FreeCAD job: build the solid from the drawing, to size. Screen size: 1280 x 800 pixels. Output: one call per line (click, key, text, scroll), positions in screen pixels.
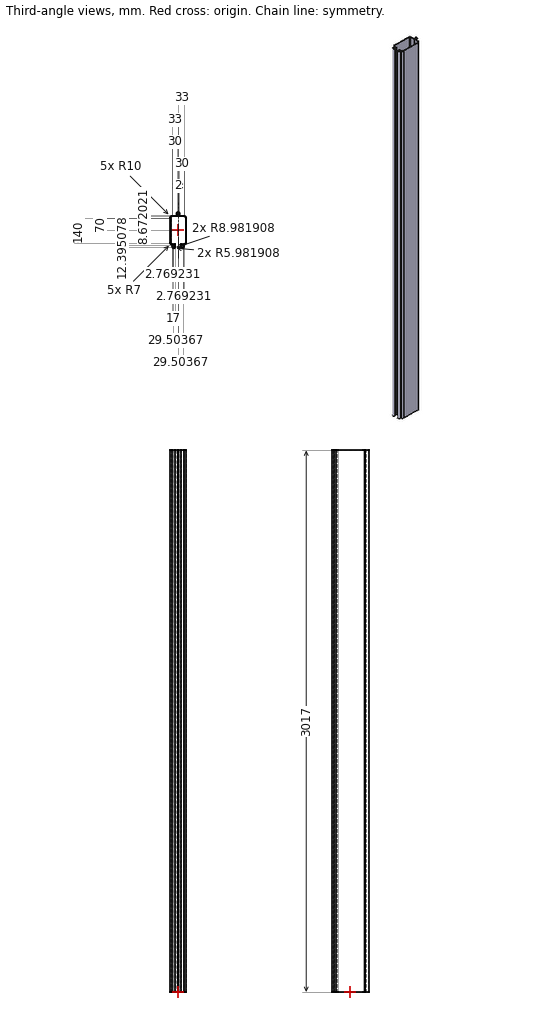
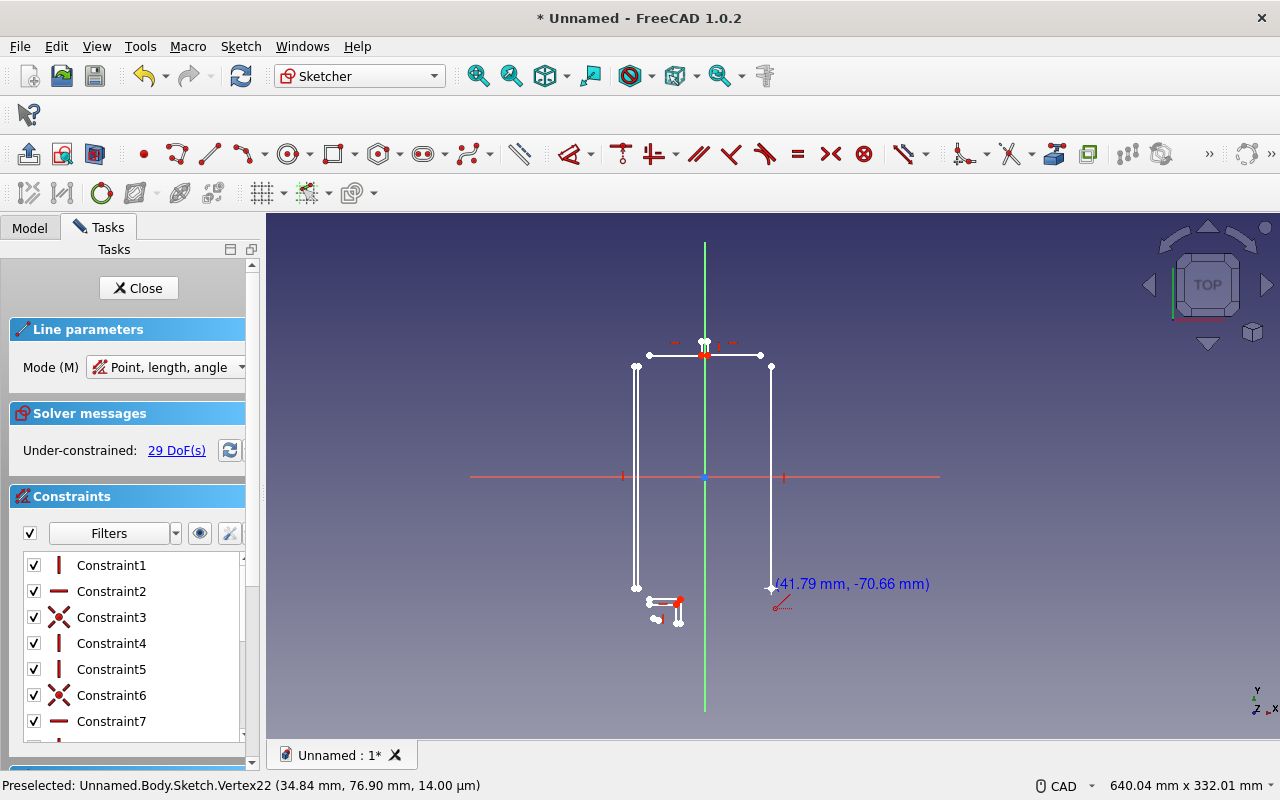
click(177, 154)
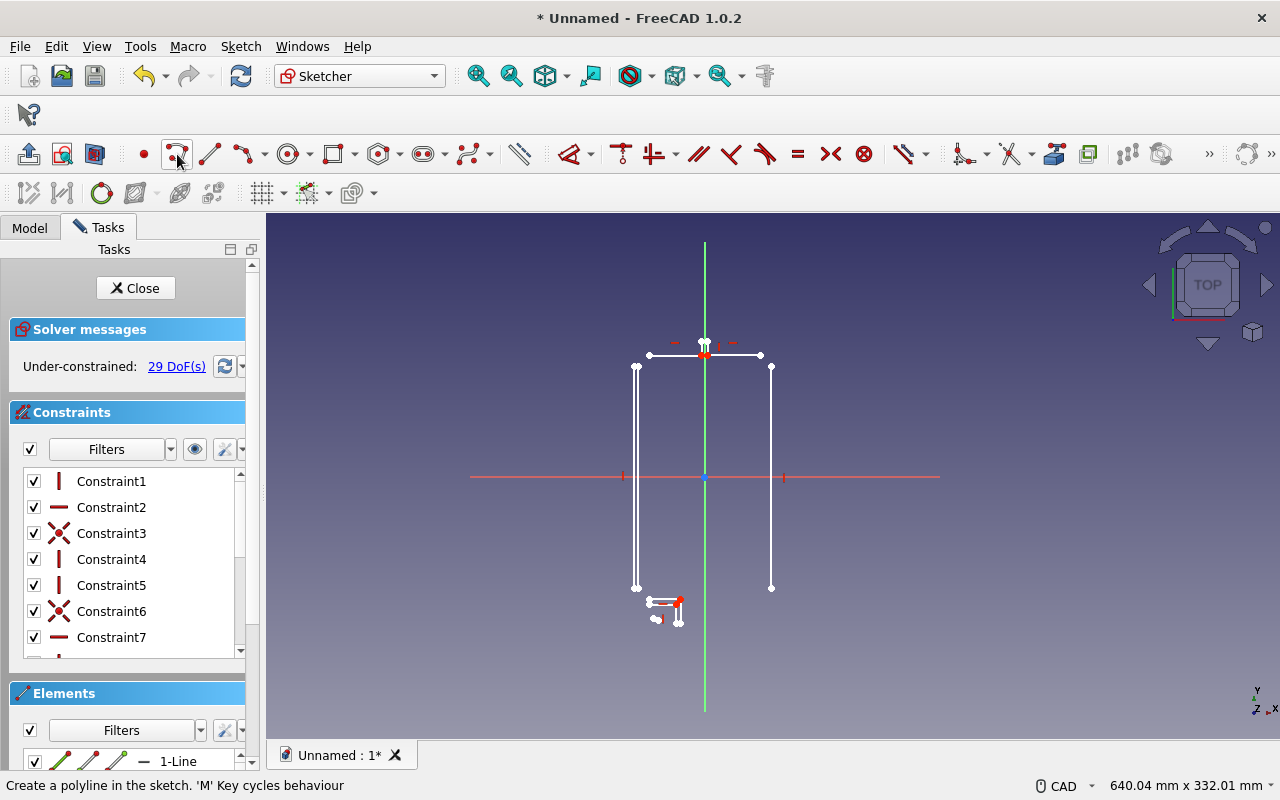
click(760, 599)
click(729, 599)
click(729, 623)
right_click(729, 623)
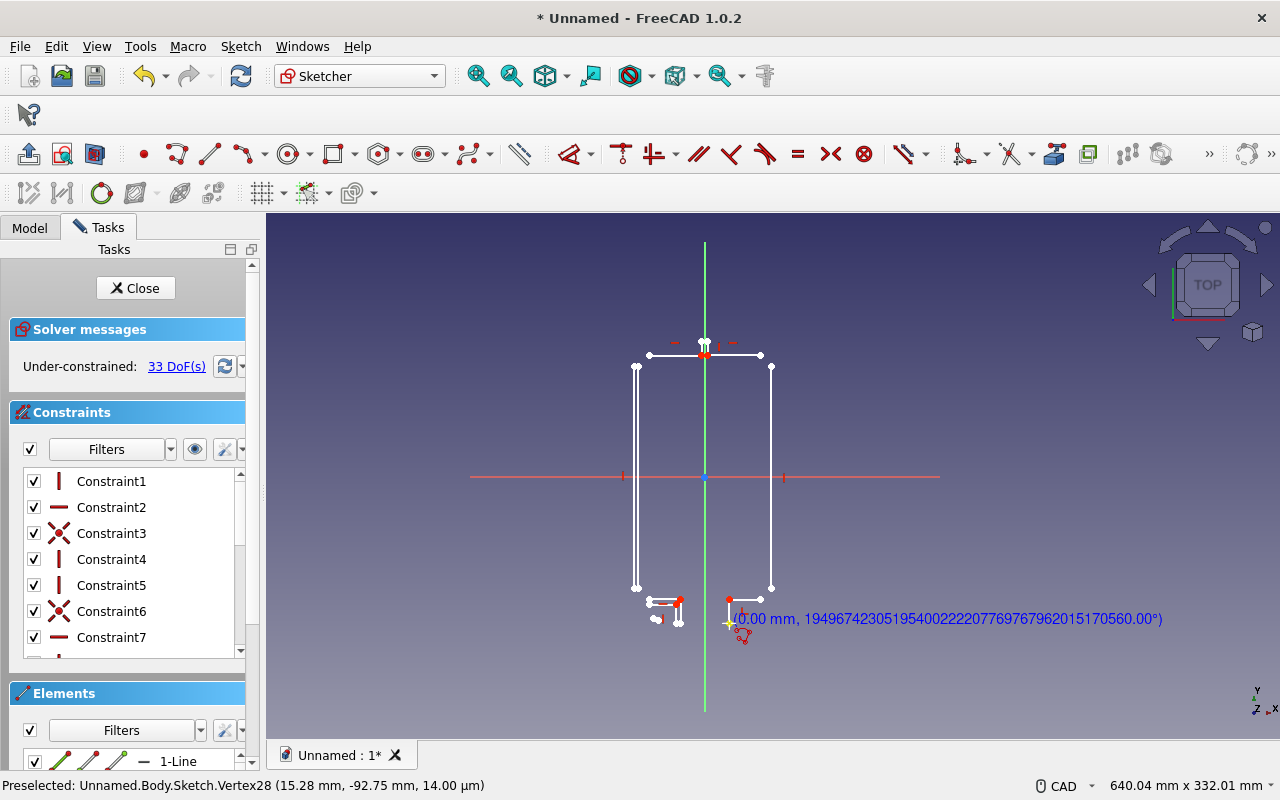
click(210, 154)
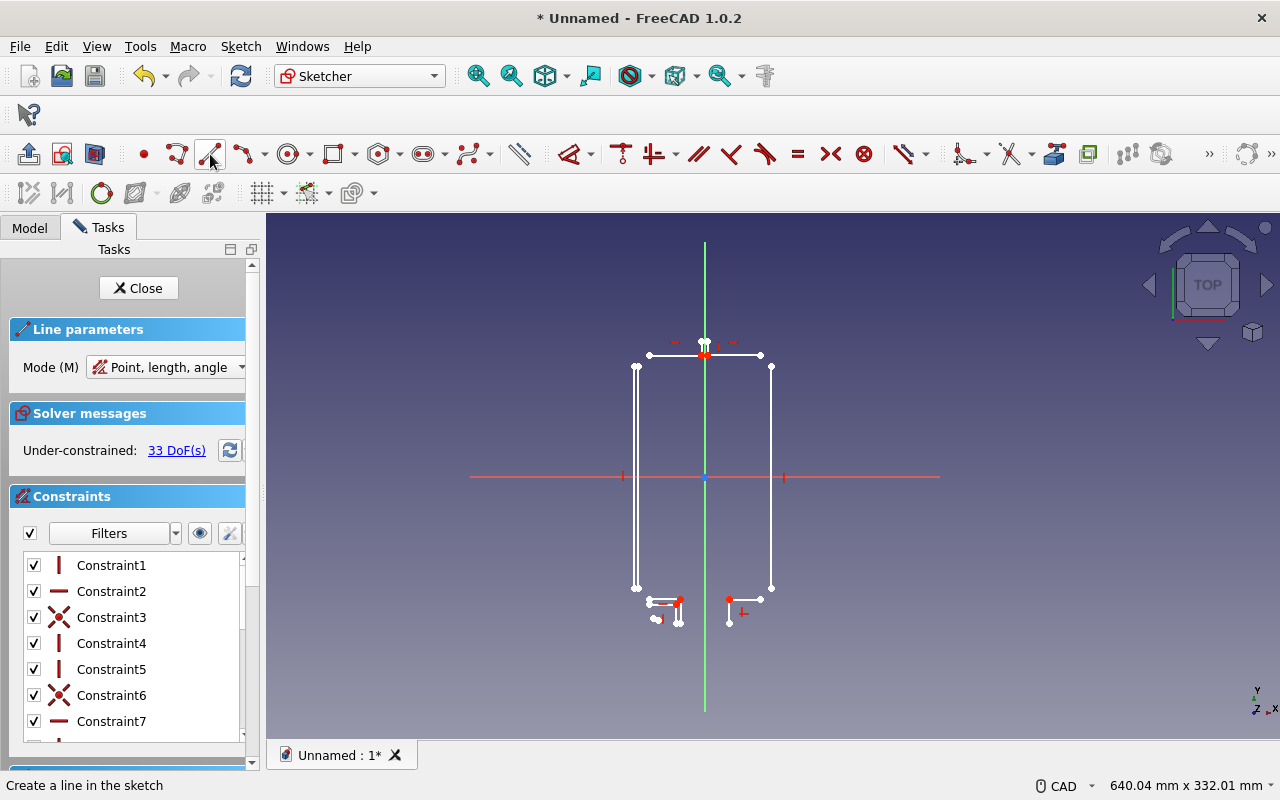
click(756, 618)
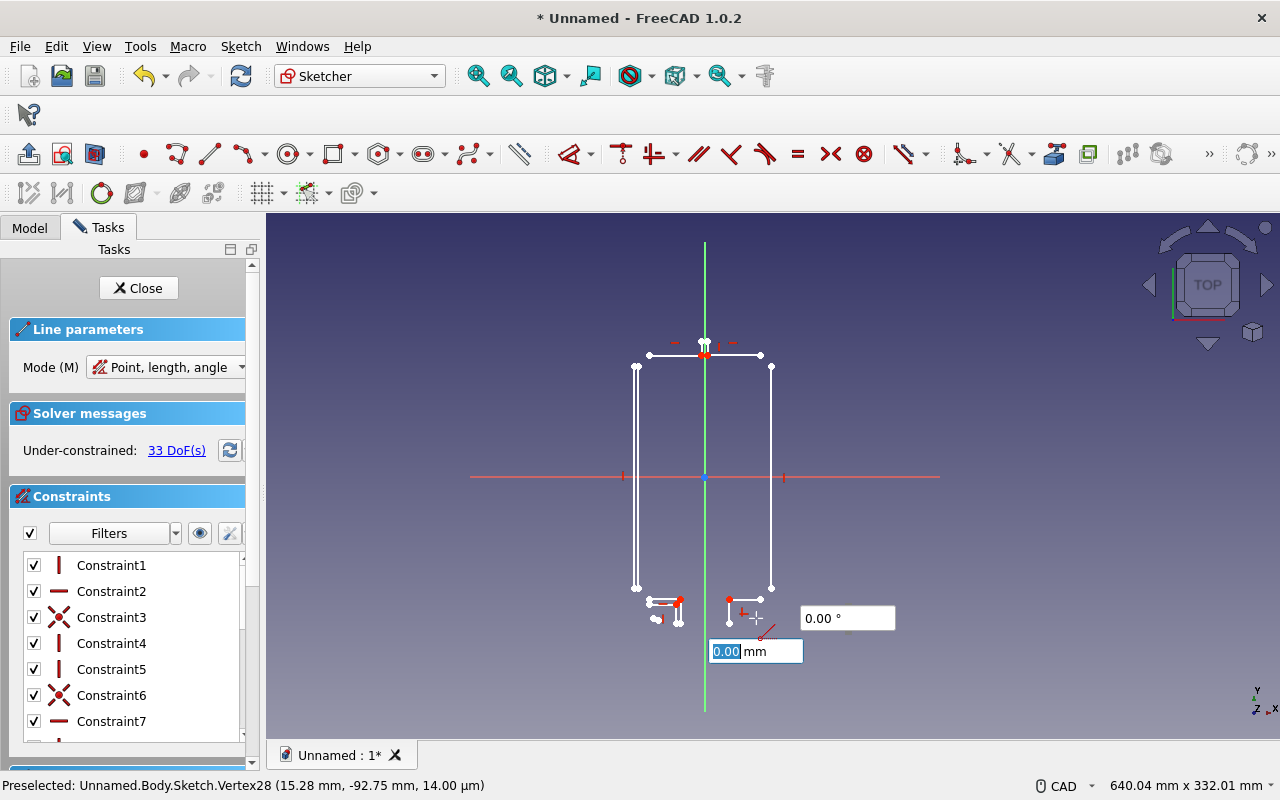
scroll(752, 620, up, 7)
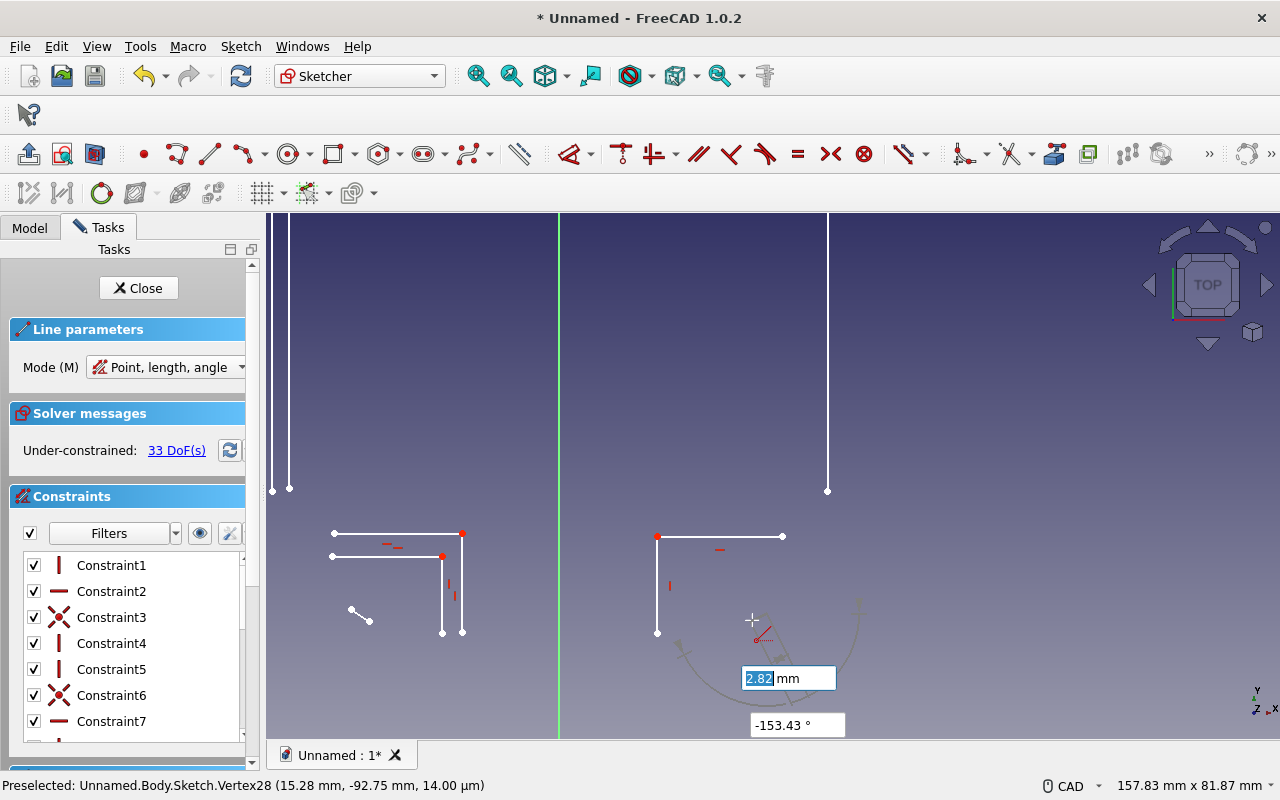
click(749, 617)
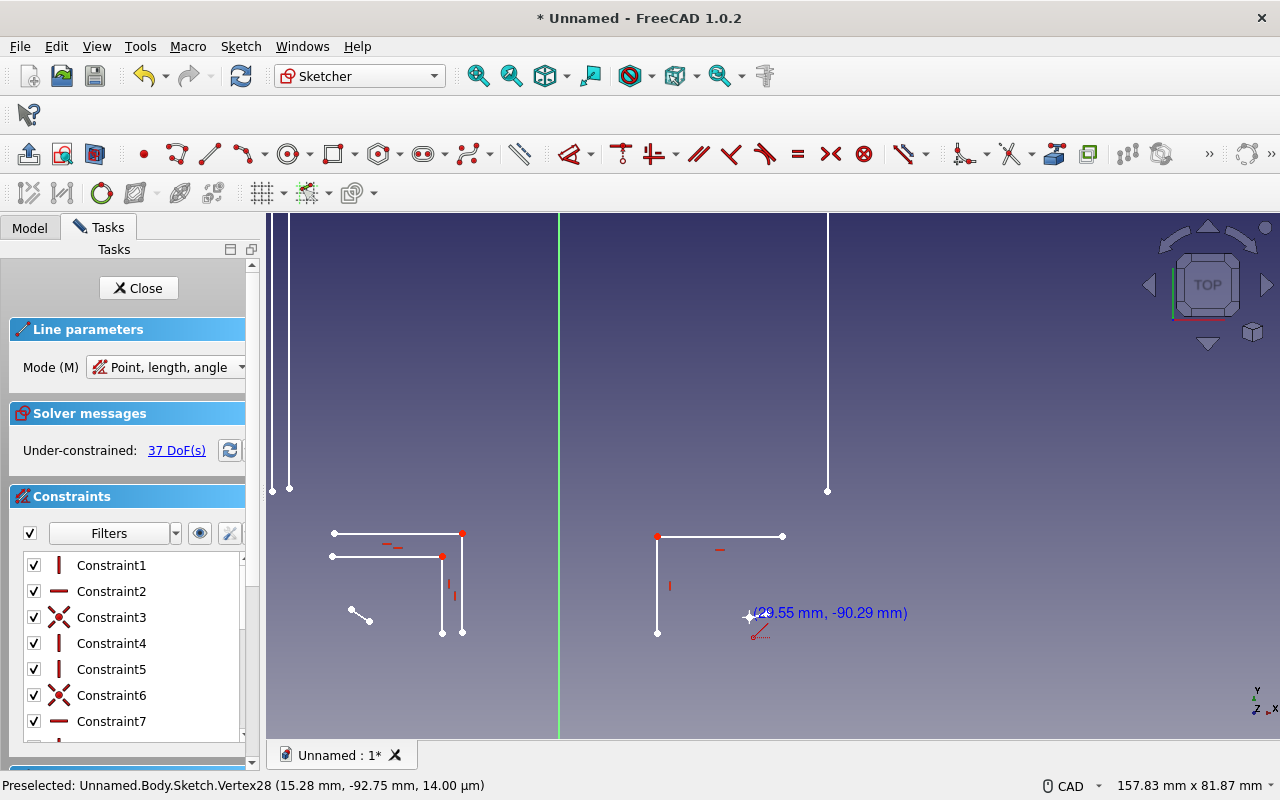
click(177, 154)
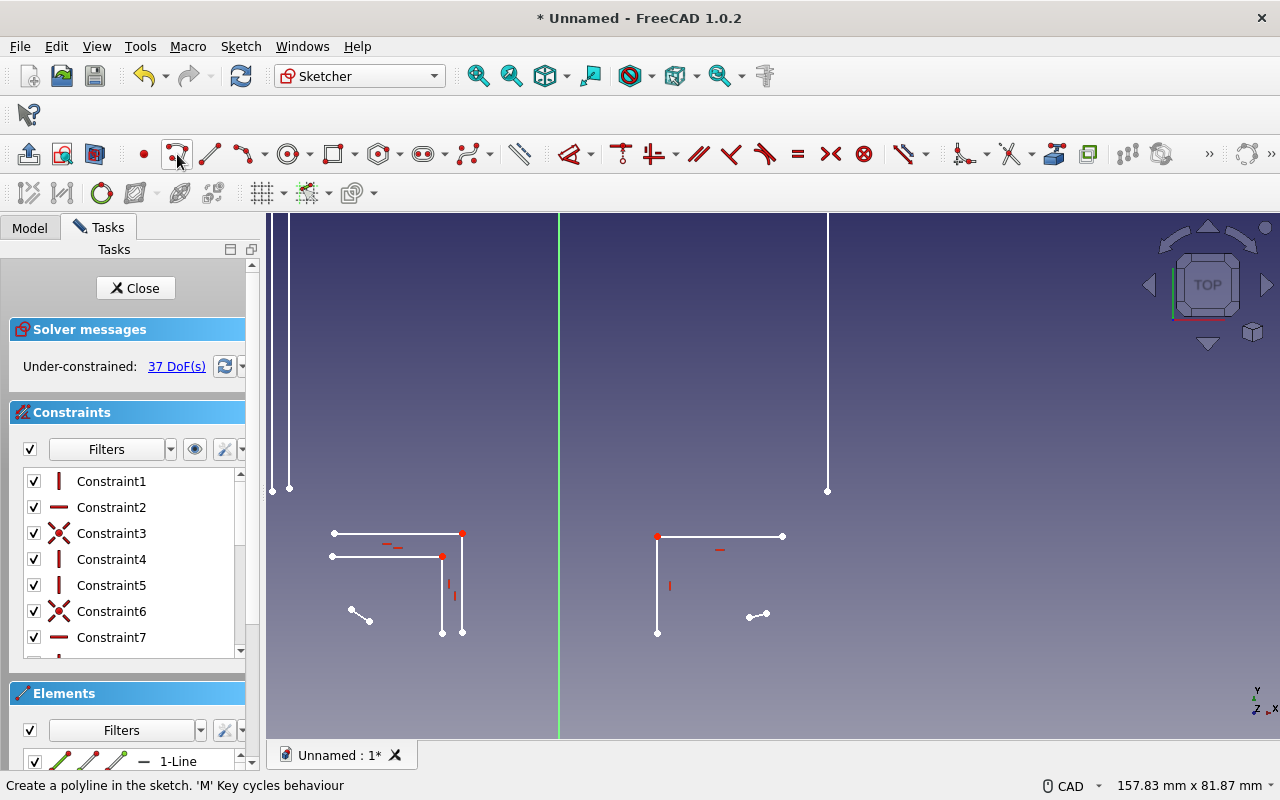
click(675, 632)
click(675, 552)
click(784, 552)
right_click(784, 552)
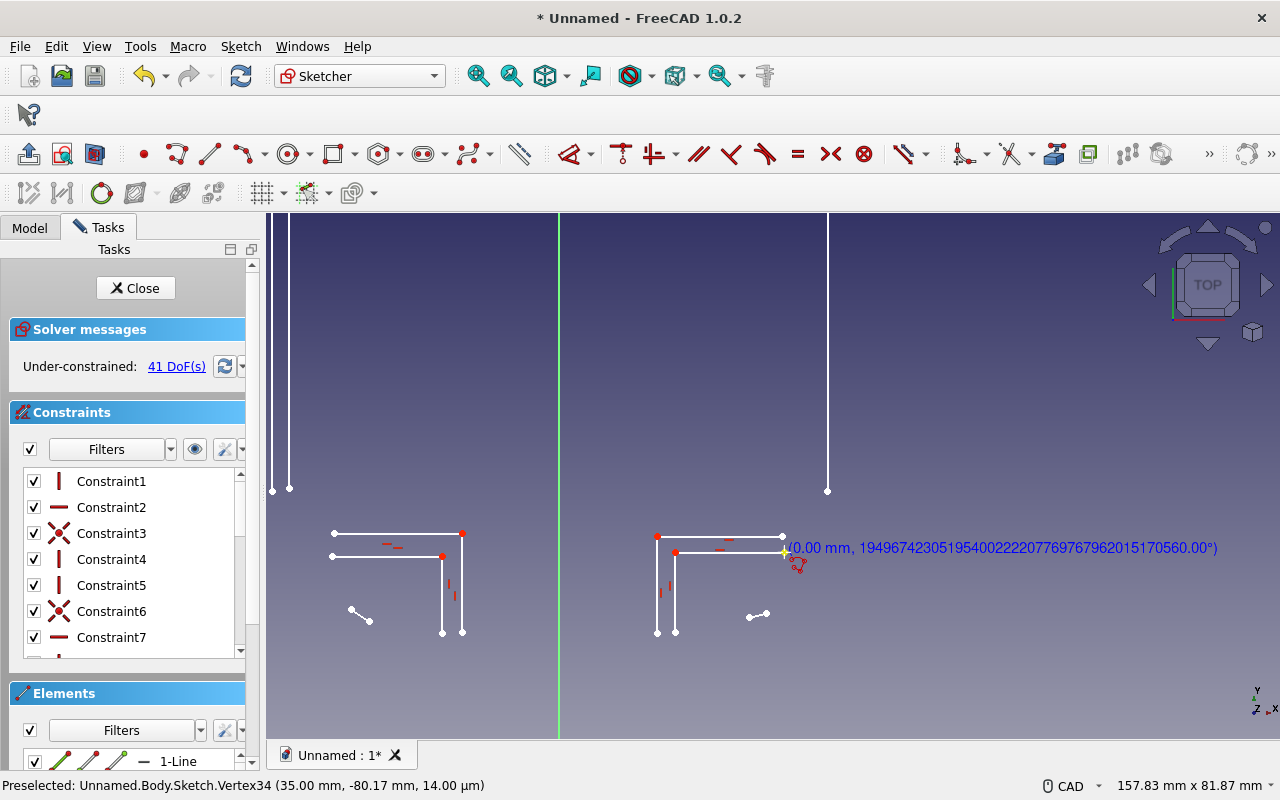
click(210, 154)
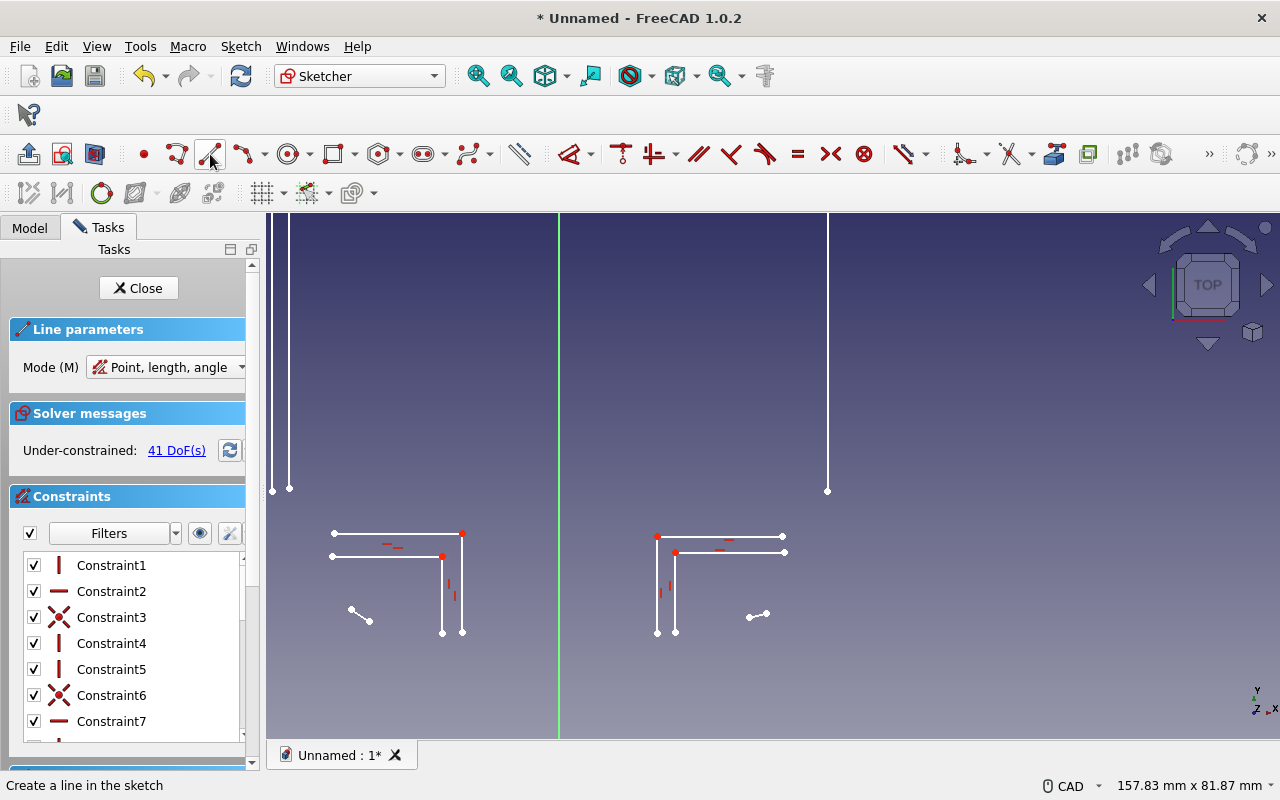
click(848, 488)